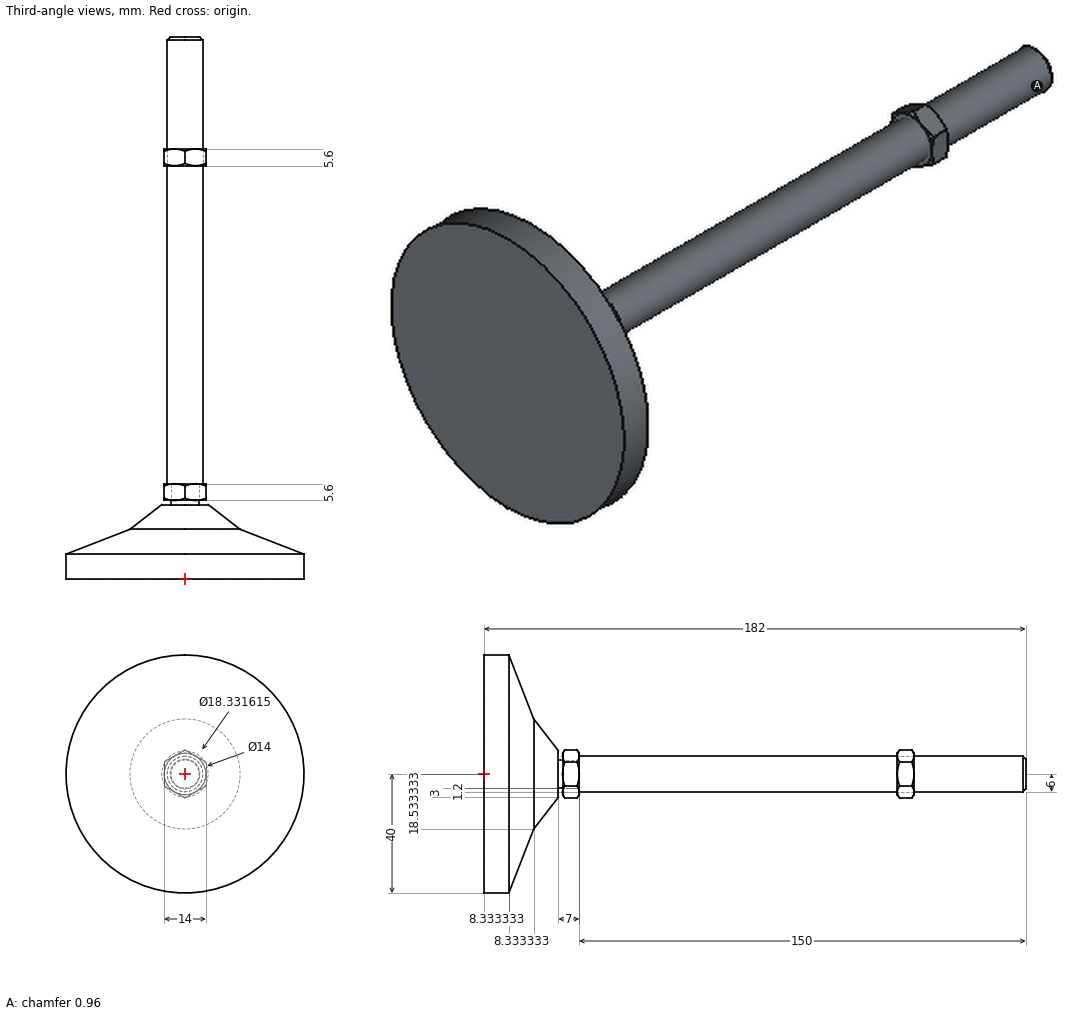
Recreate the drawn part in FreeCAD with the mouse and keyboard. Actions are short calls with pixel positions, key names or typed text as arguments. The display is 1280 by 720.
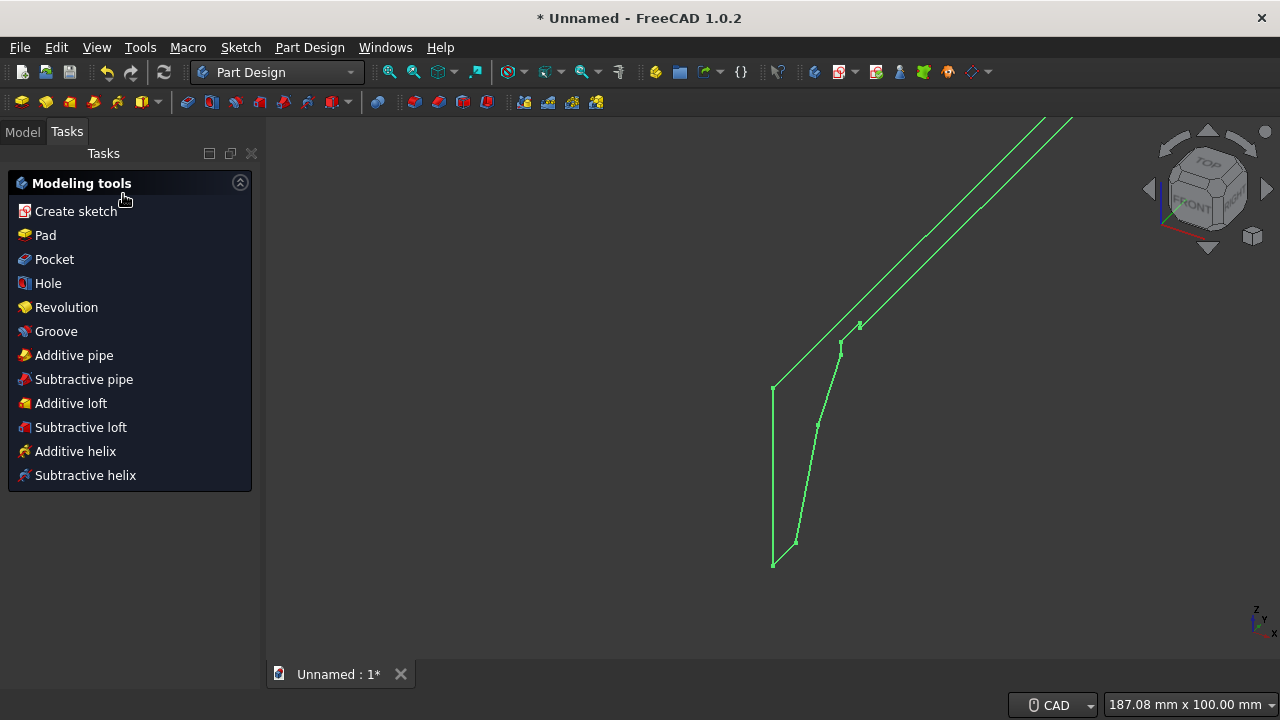
click(46, 102)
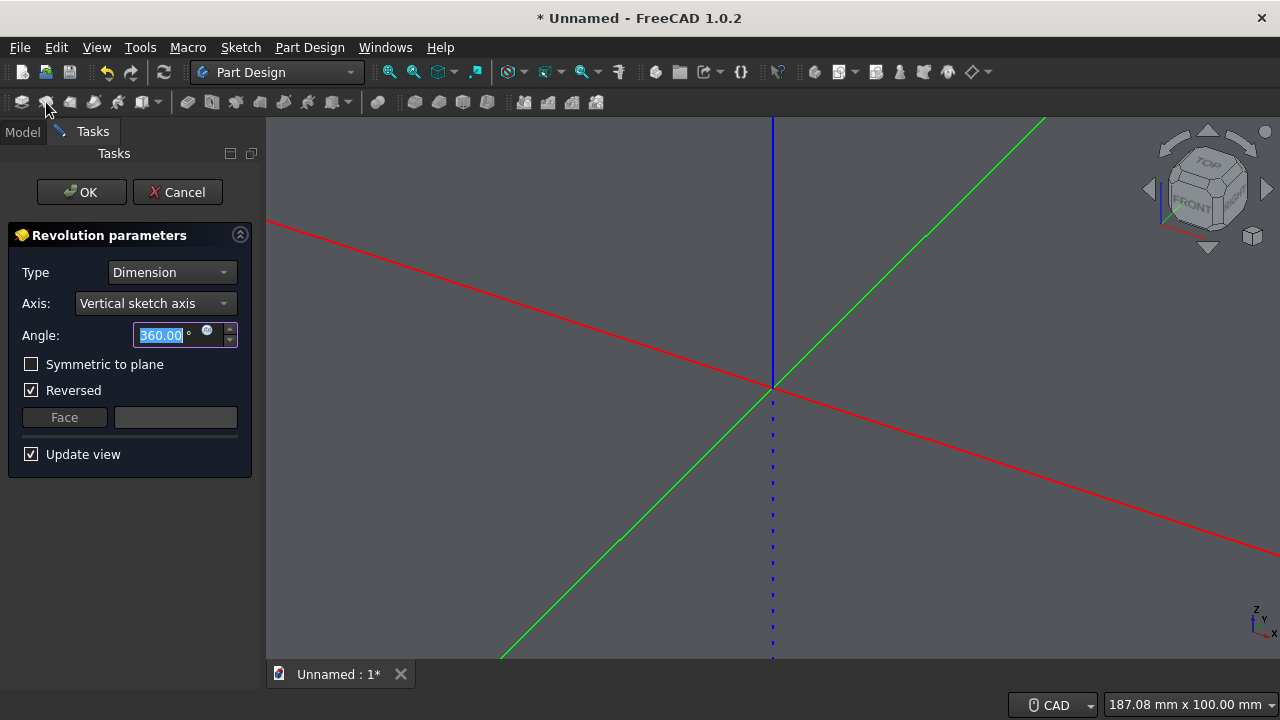
click(156, 304)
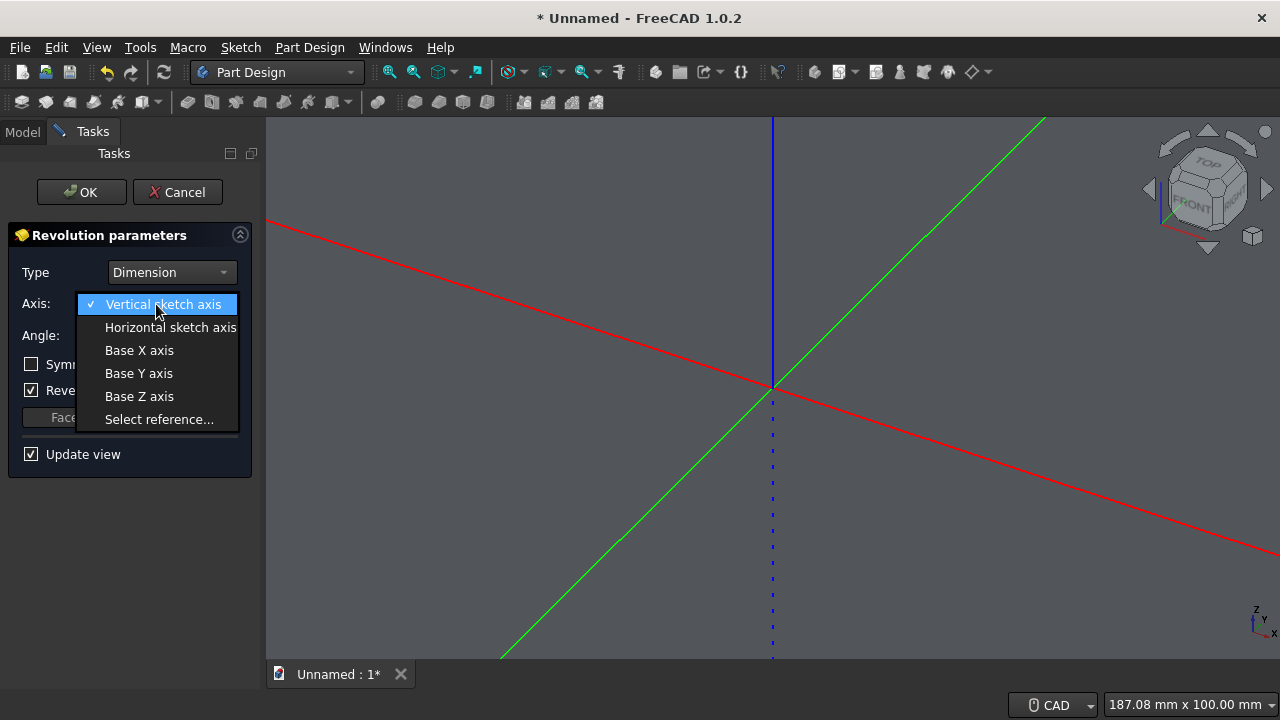
click(156, 328)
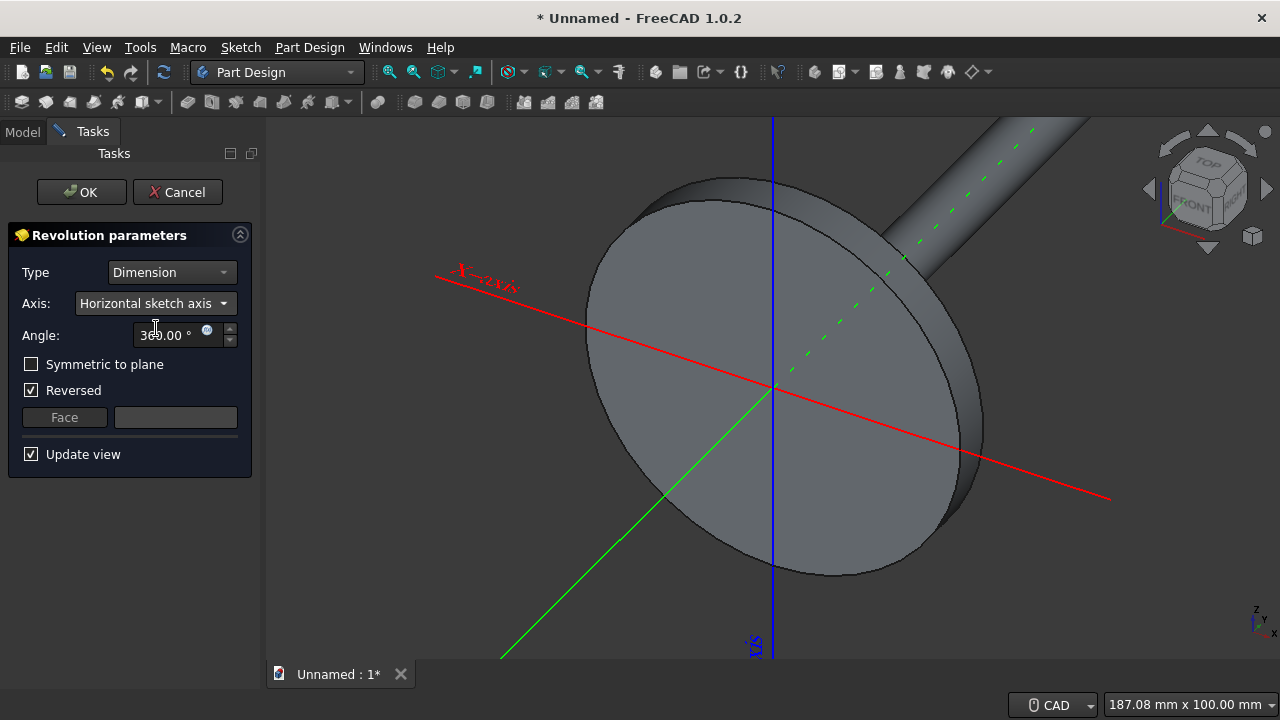
click(82, 192)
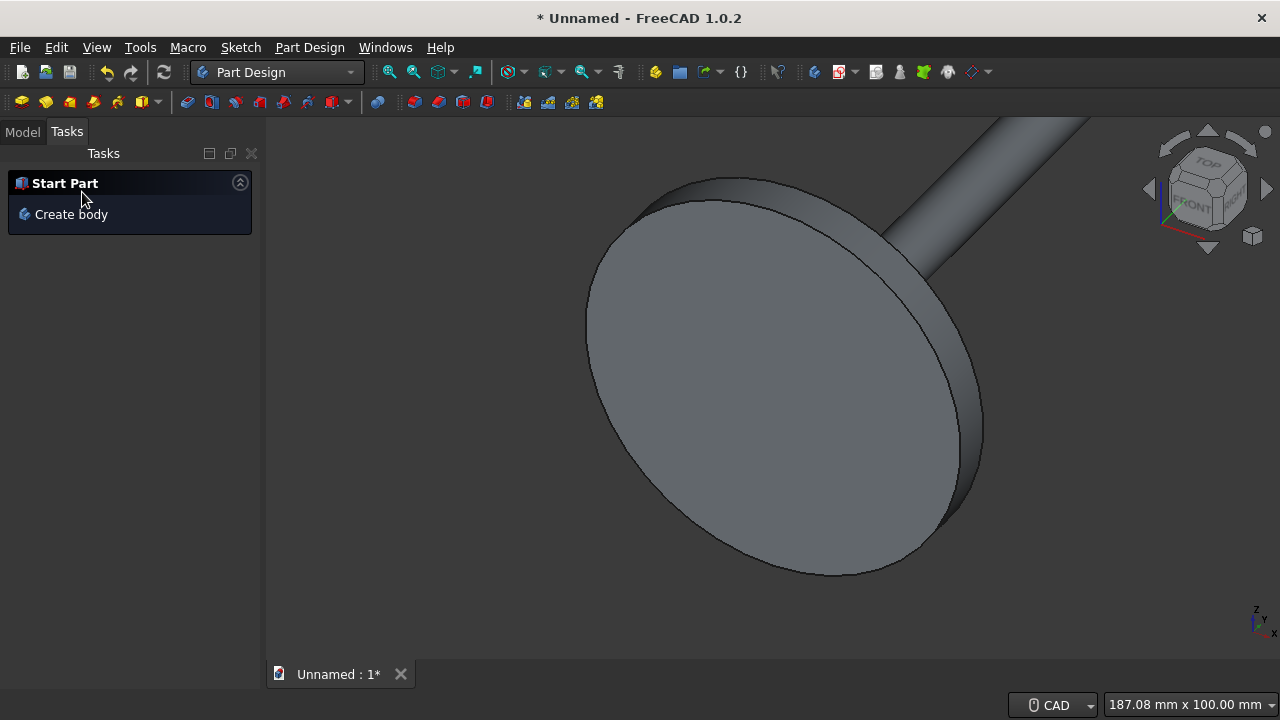
click(390, 72)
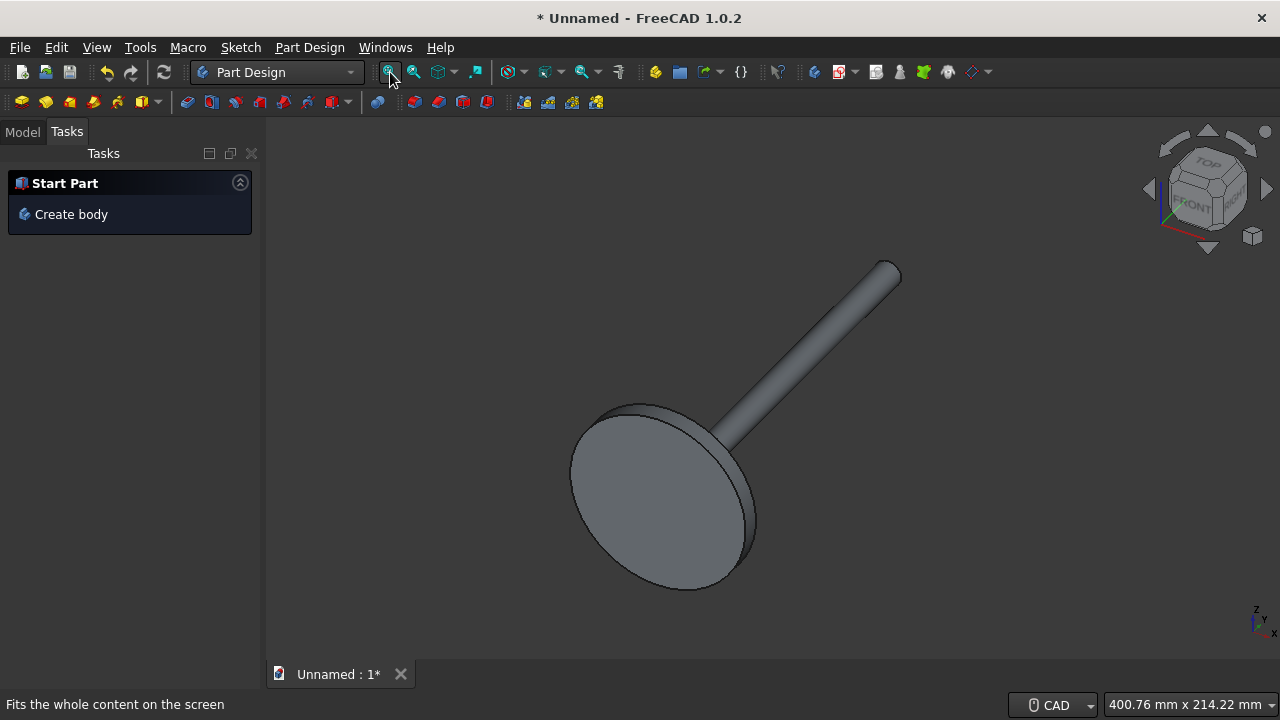
click(888, 260)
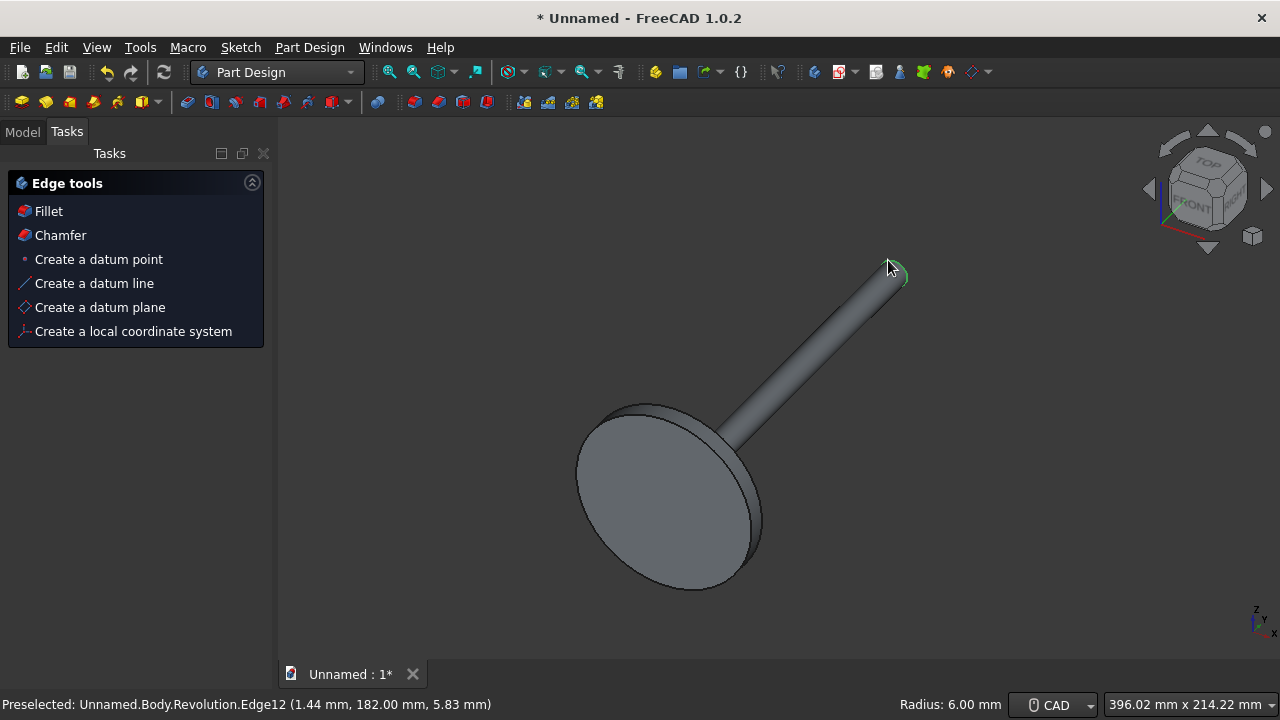
click(440, 102)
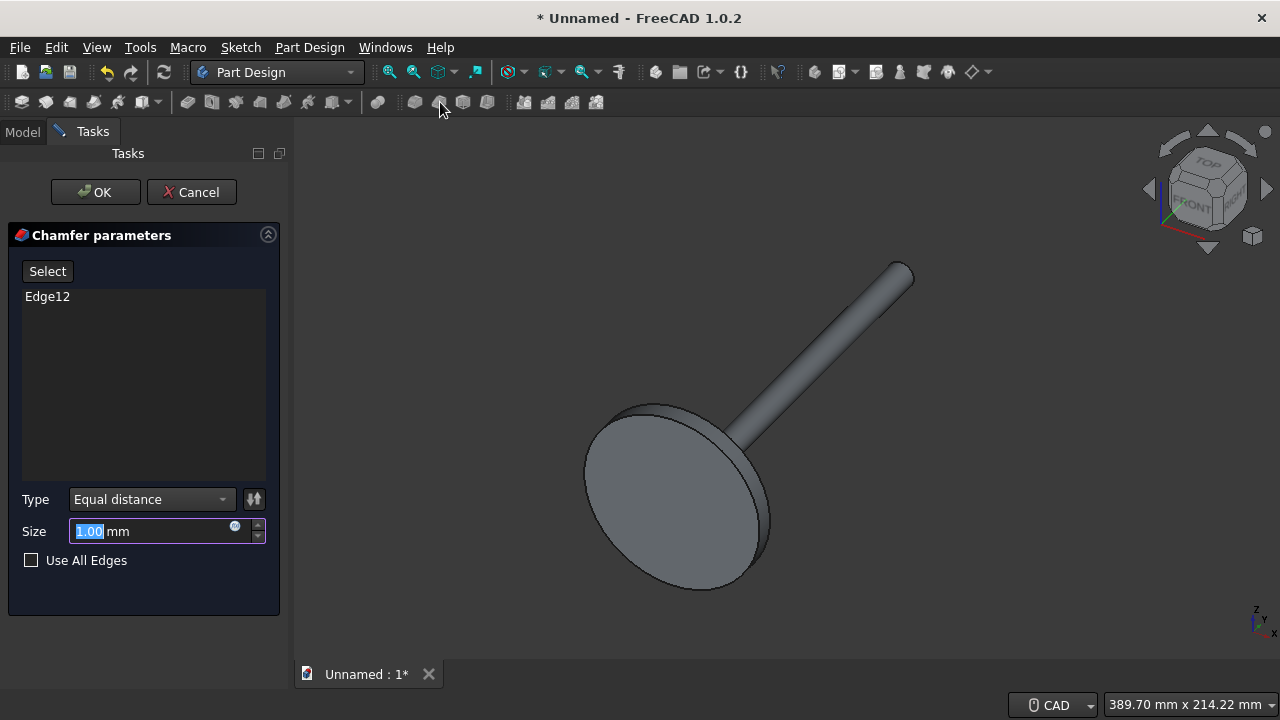
text(0.96)
key(Tab)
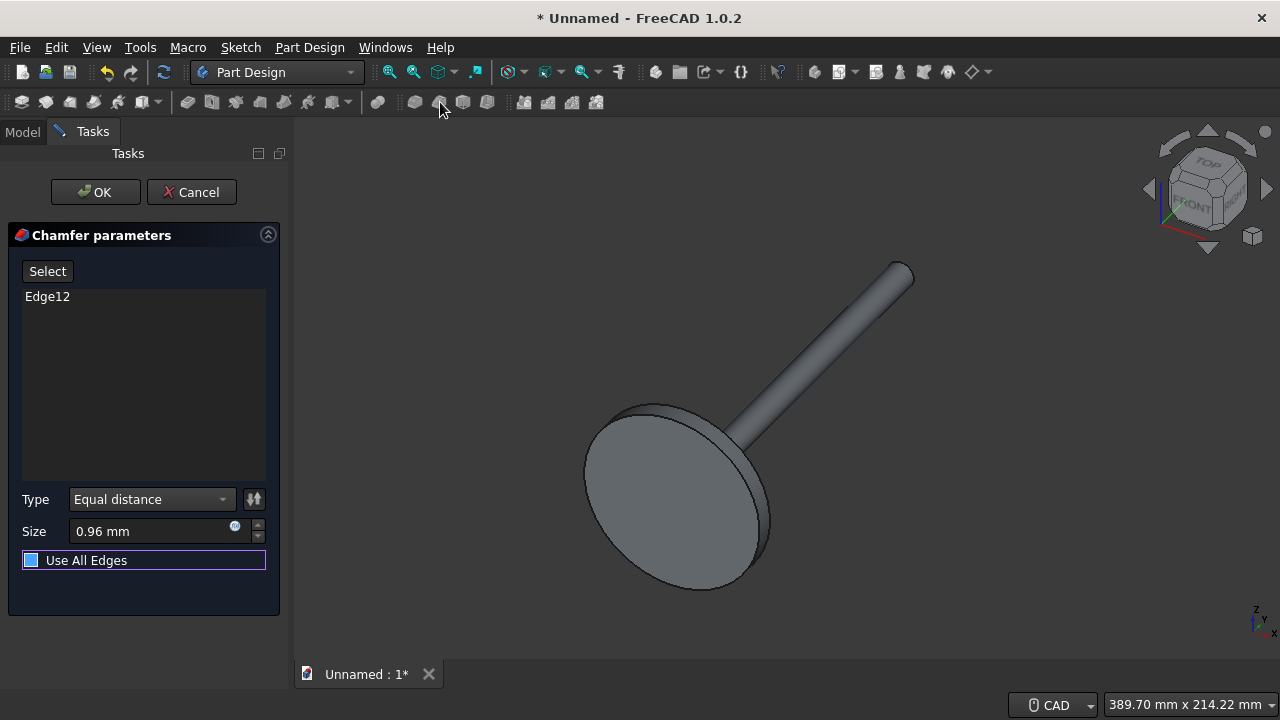
click(96, 192)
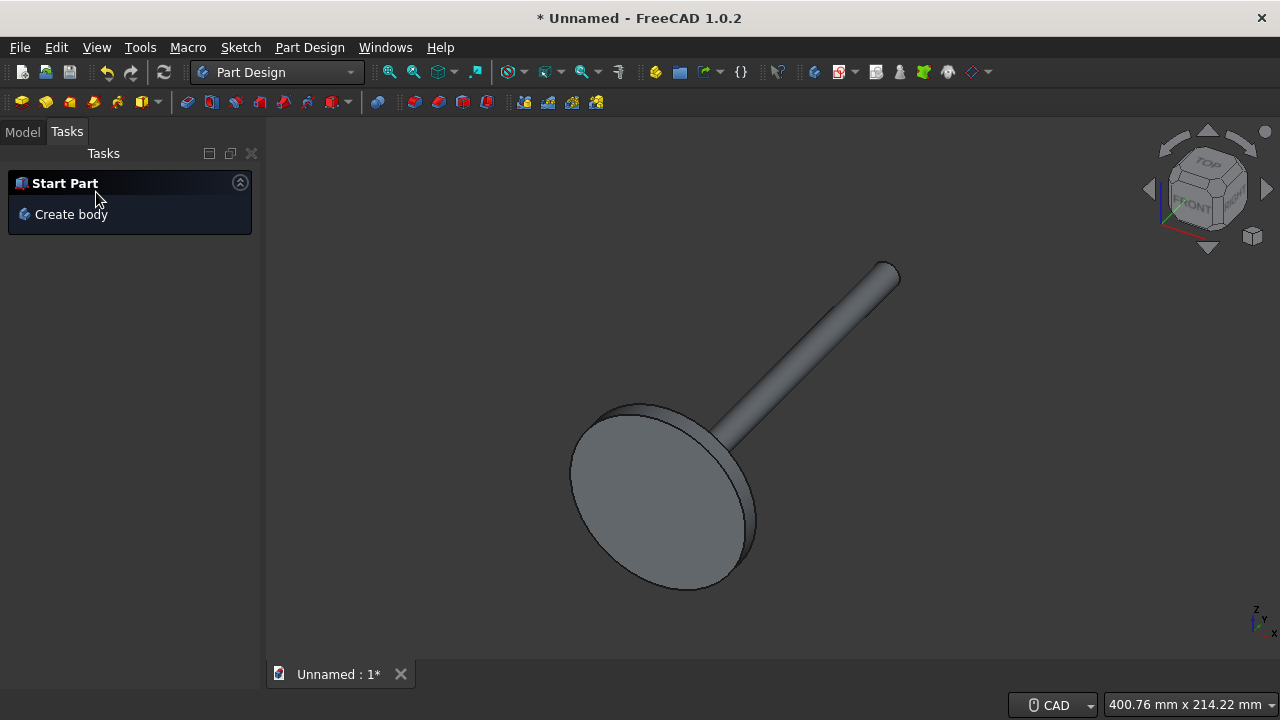
click(816, 72)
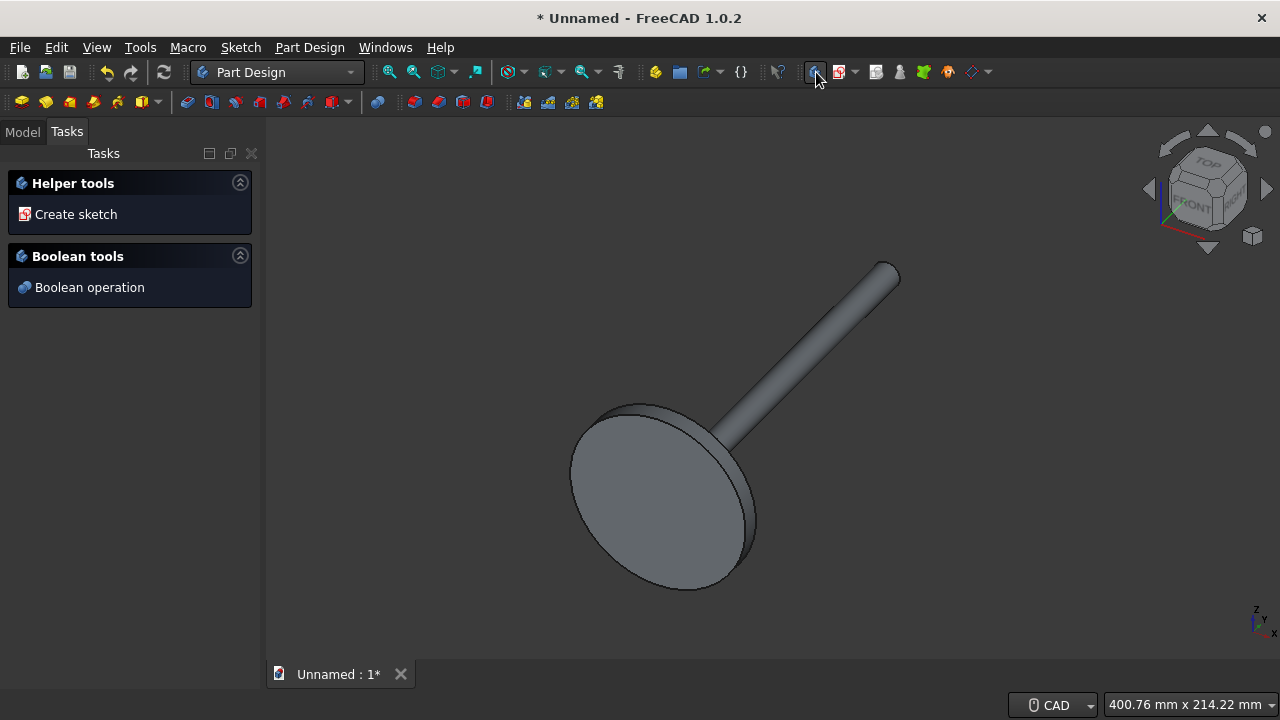
click(23, 131)